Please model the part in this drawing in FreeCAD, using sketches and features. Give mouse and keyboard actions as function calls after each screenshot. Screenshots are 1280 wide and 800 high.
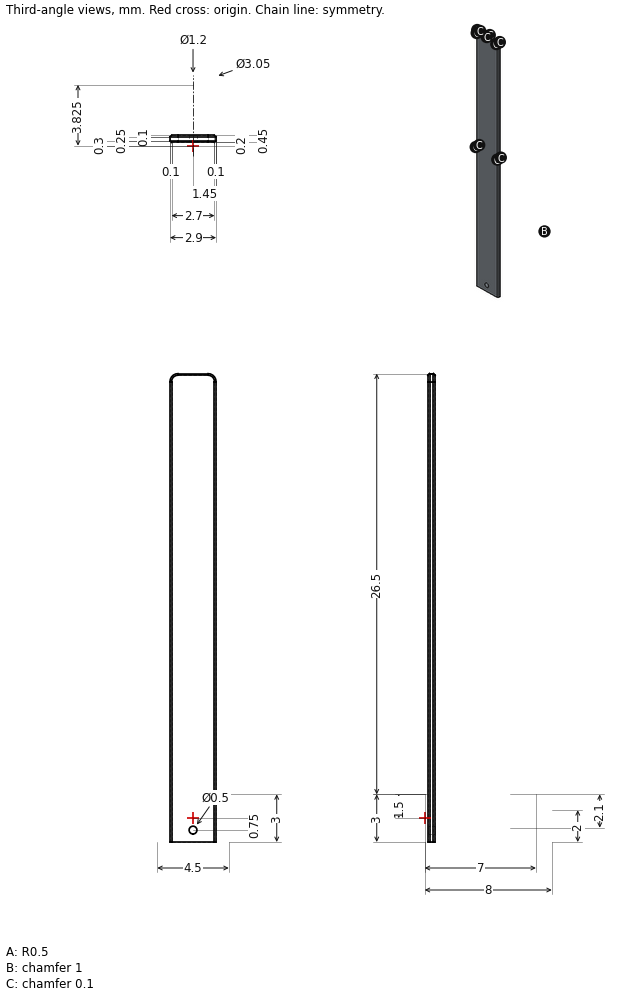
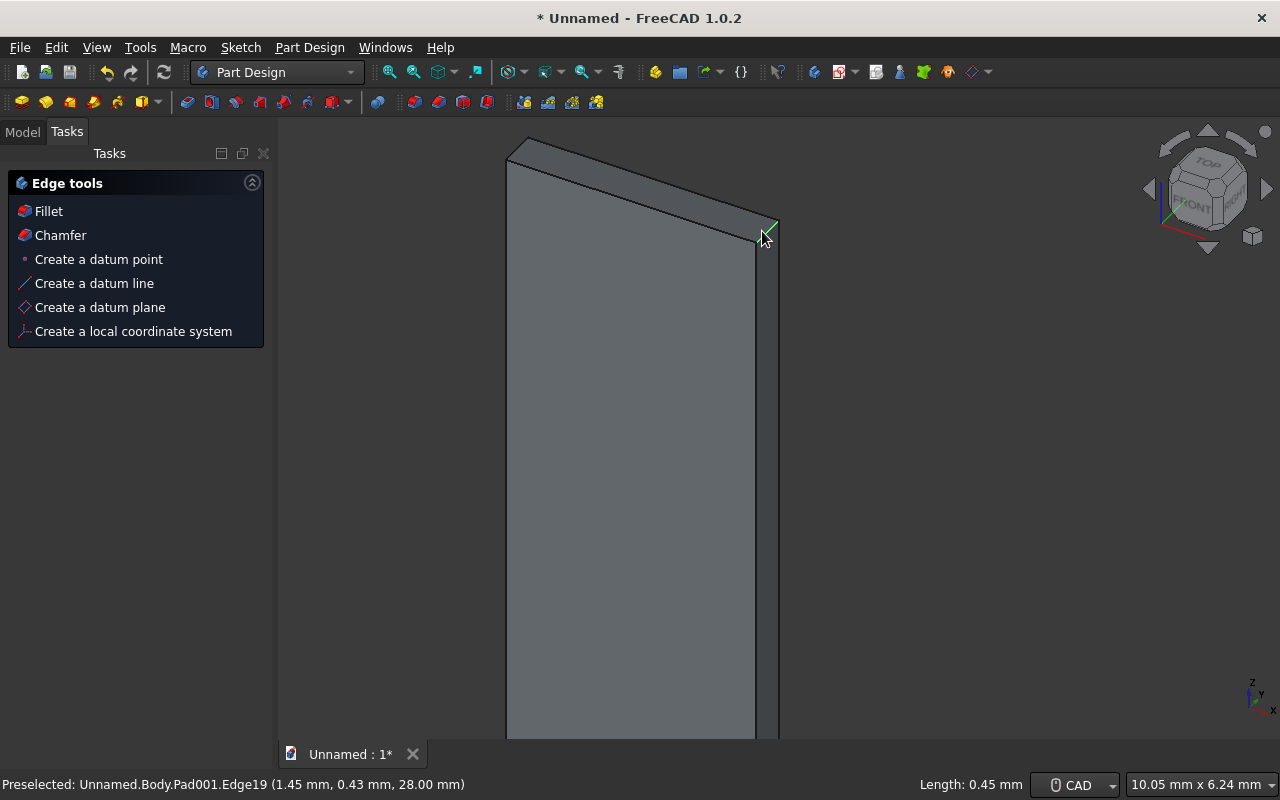
key(v)
key(f)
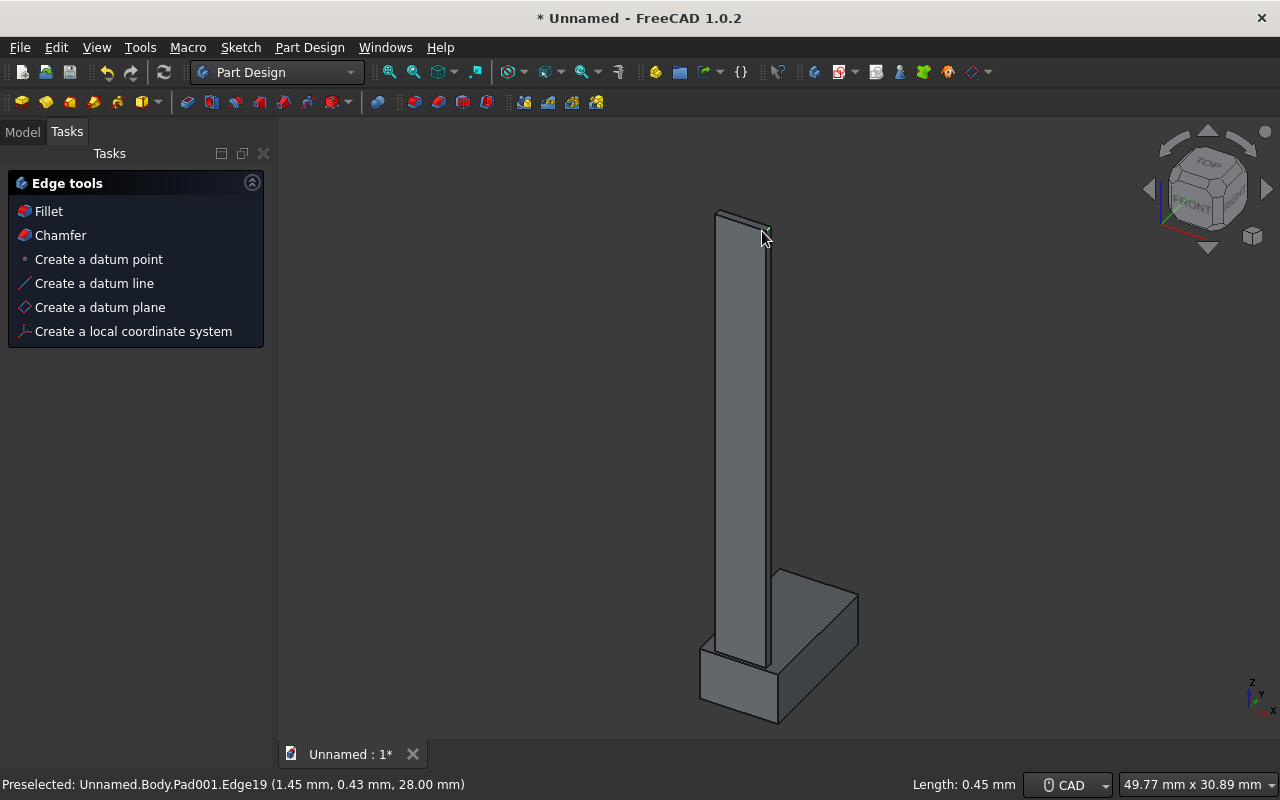
key(0)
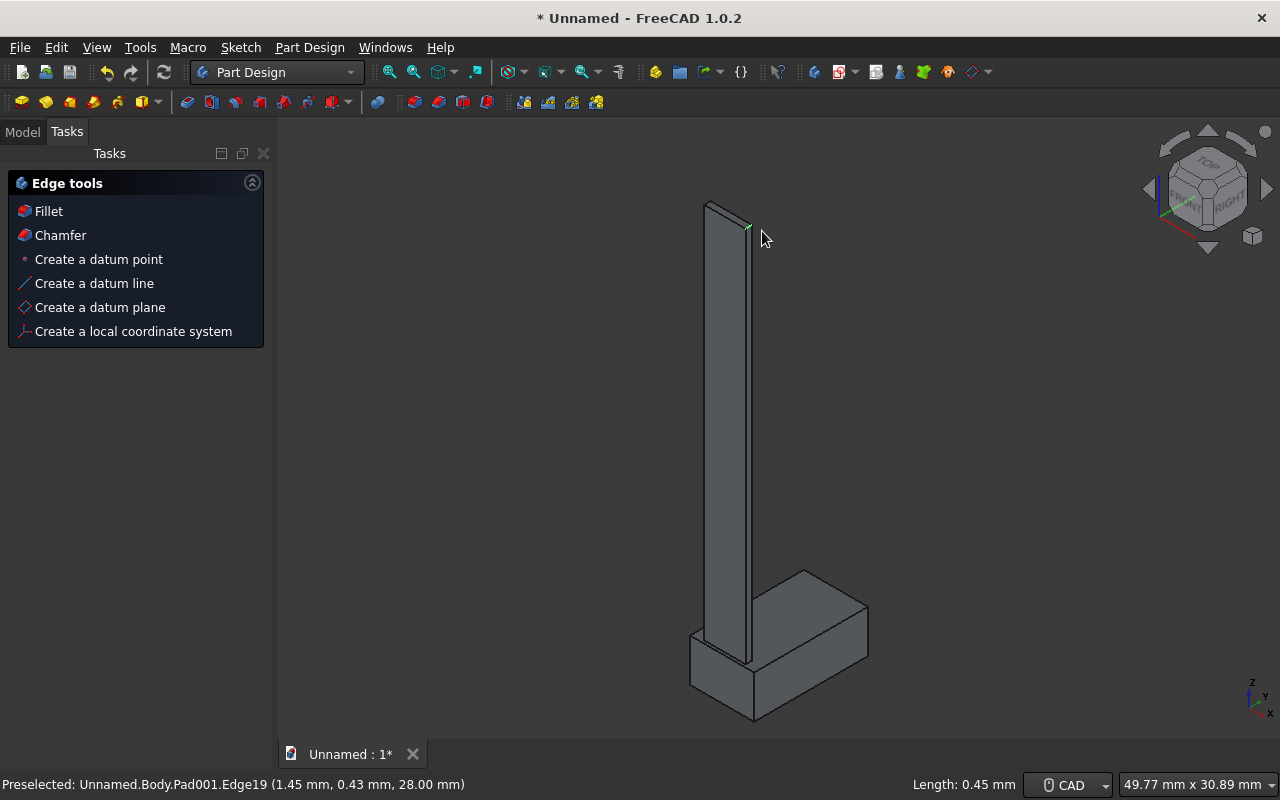
scroll(707, 202, up, 8)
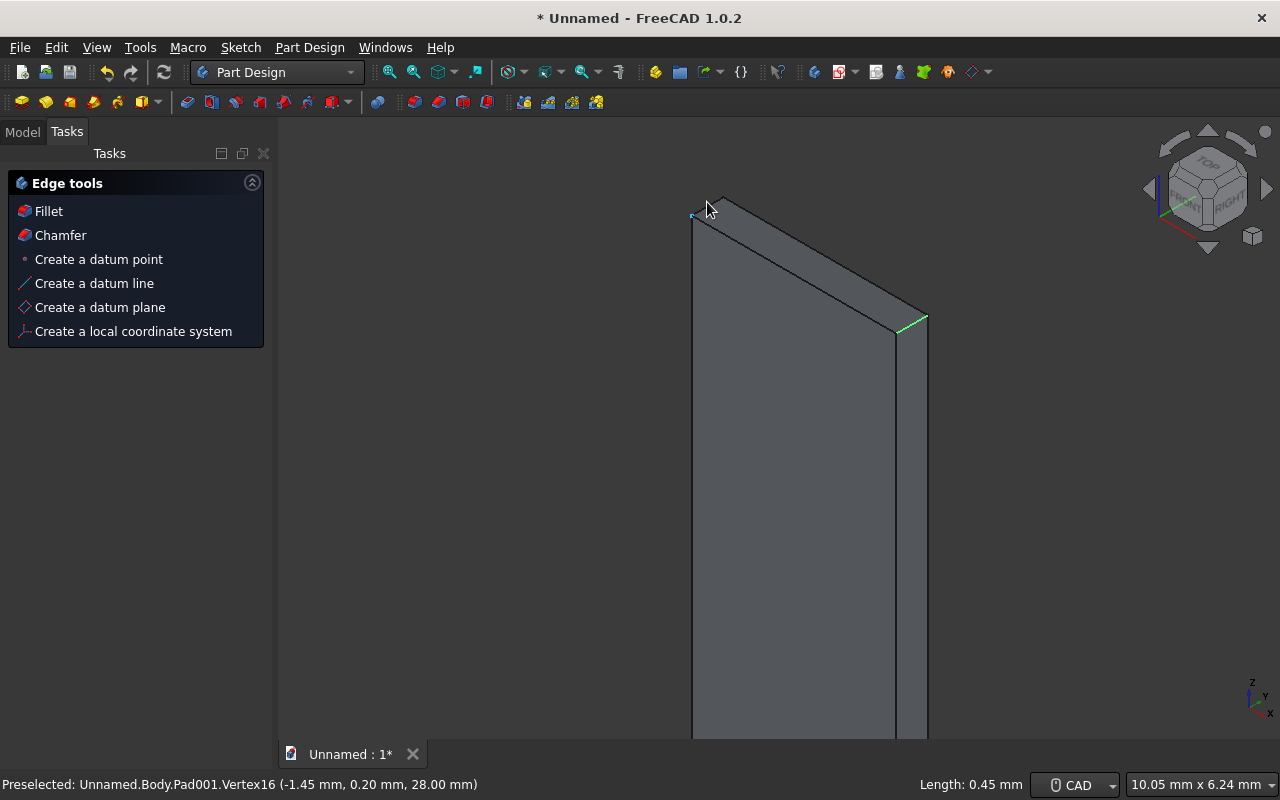
key(v)
key(f)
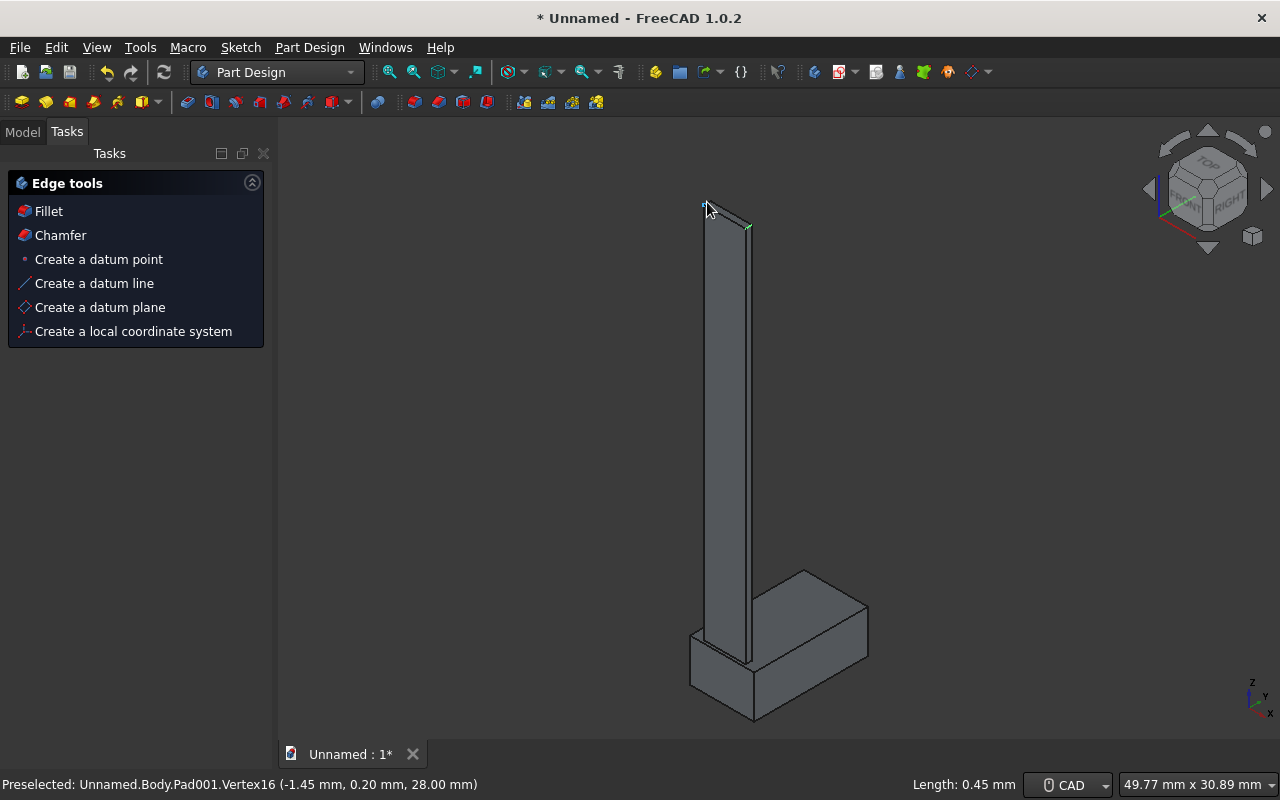
key(2)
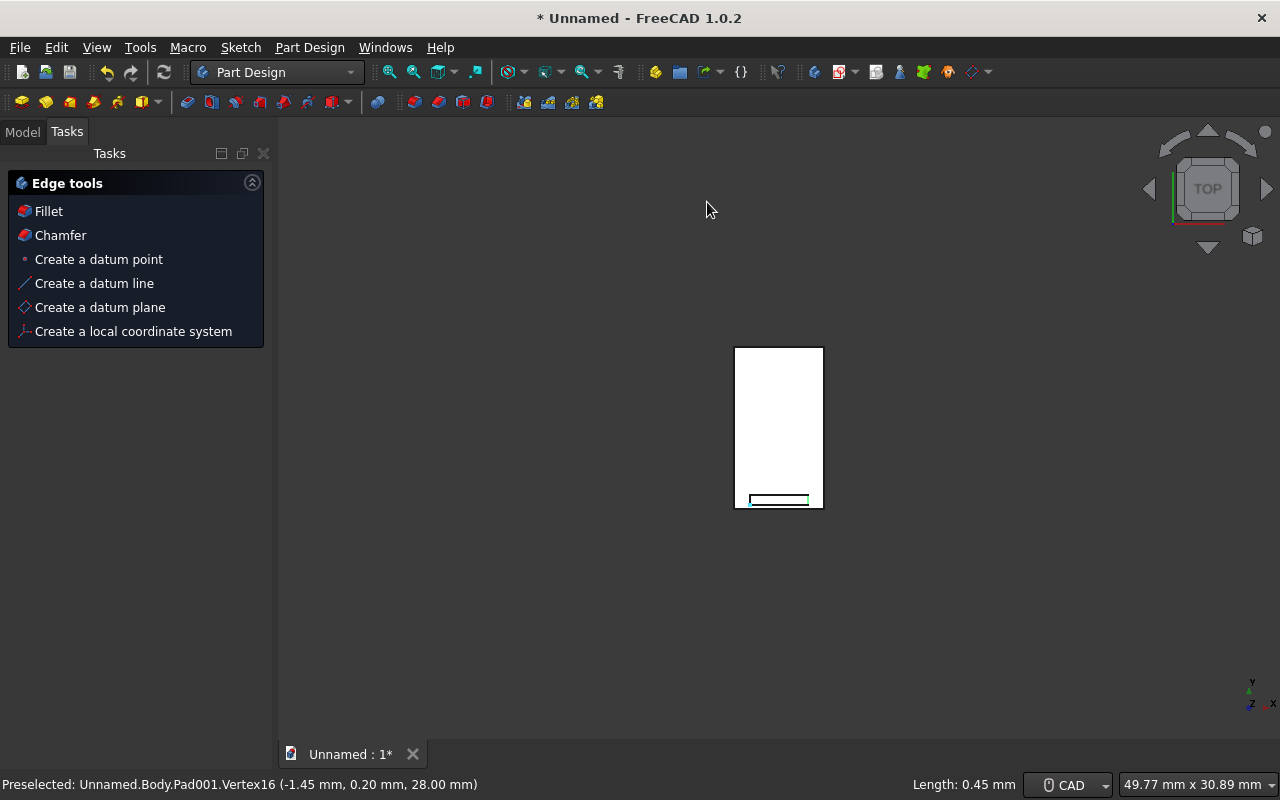
click(390, 72)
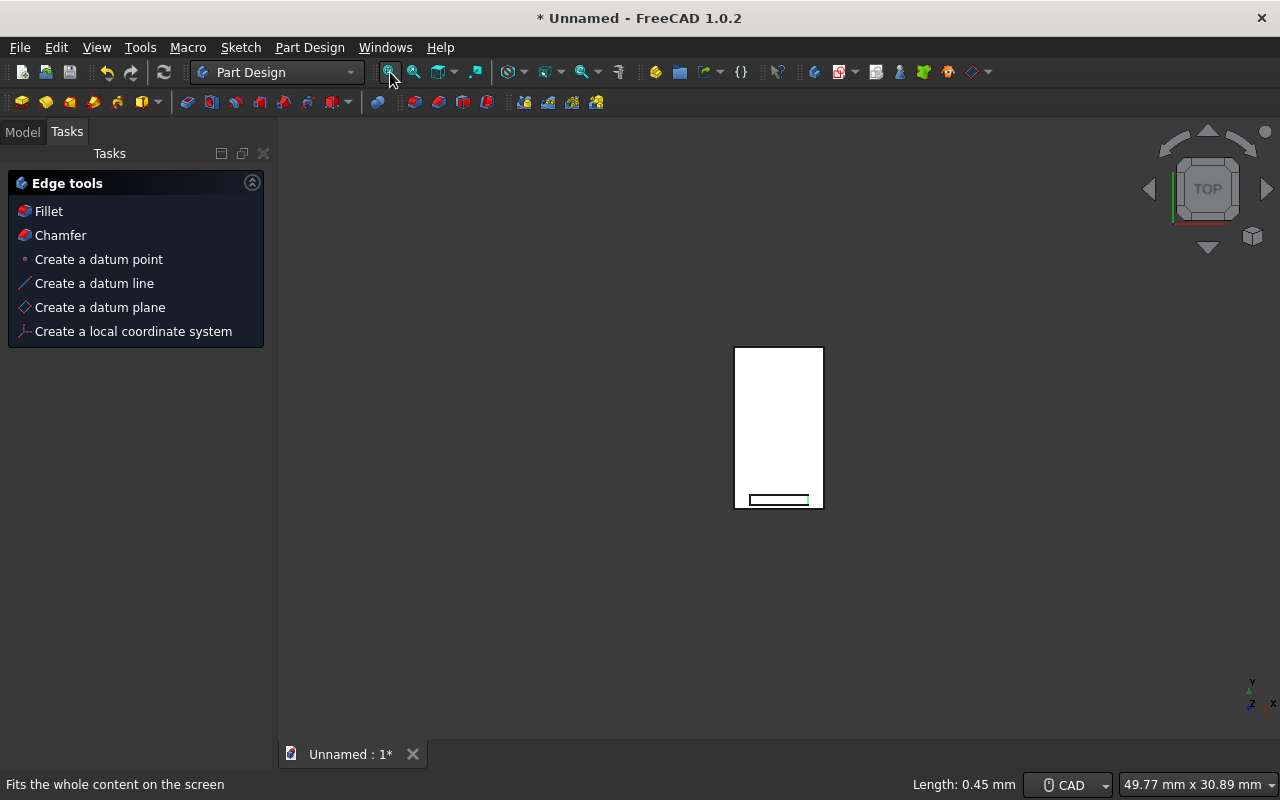
scroll(750, 499, up, 8)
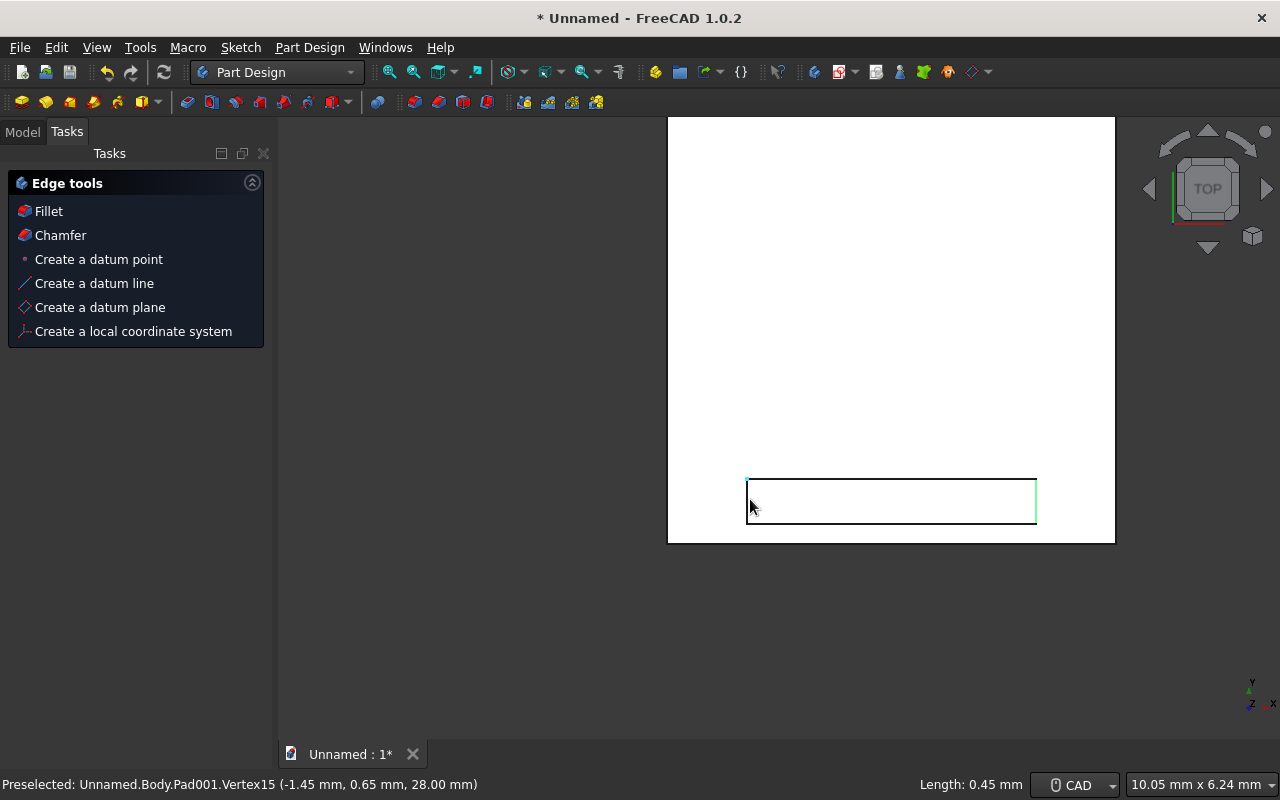
click(747, 500, ctrl)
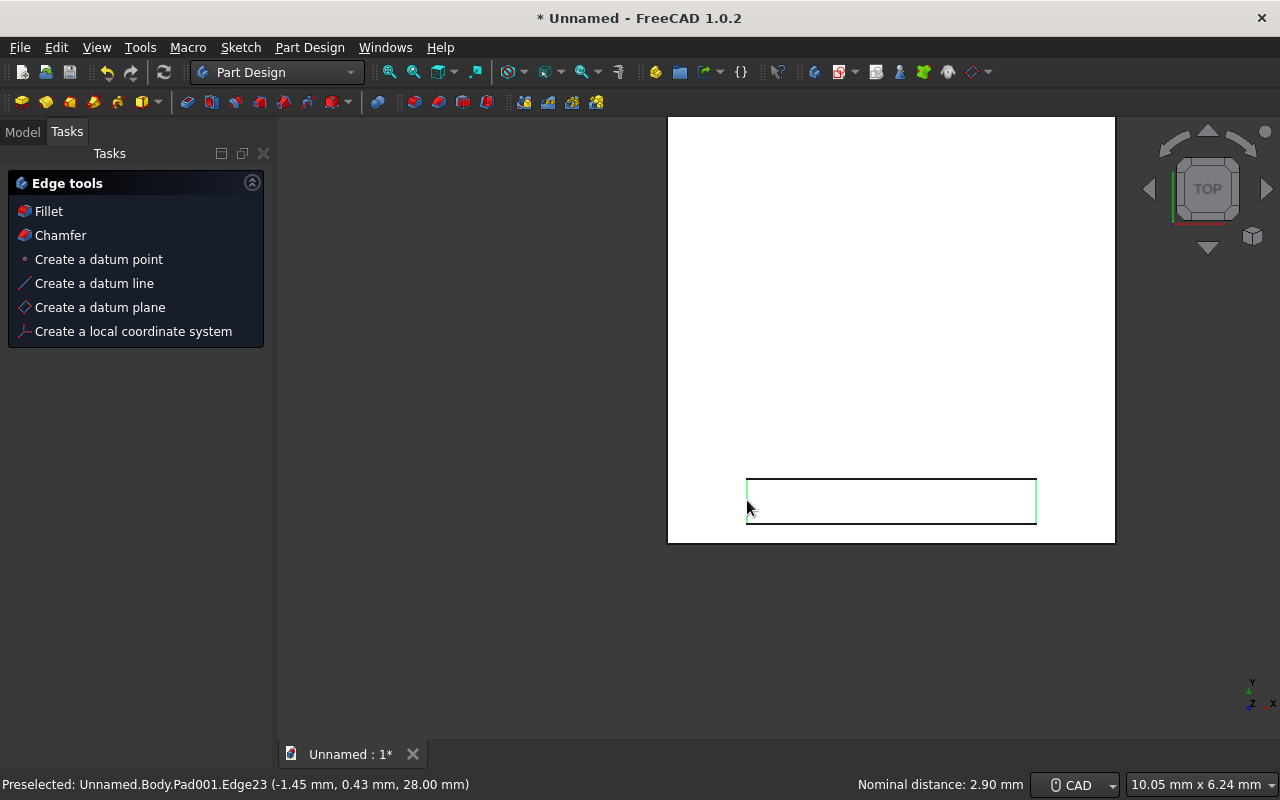
click(416, 102)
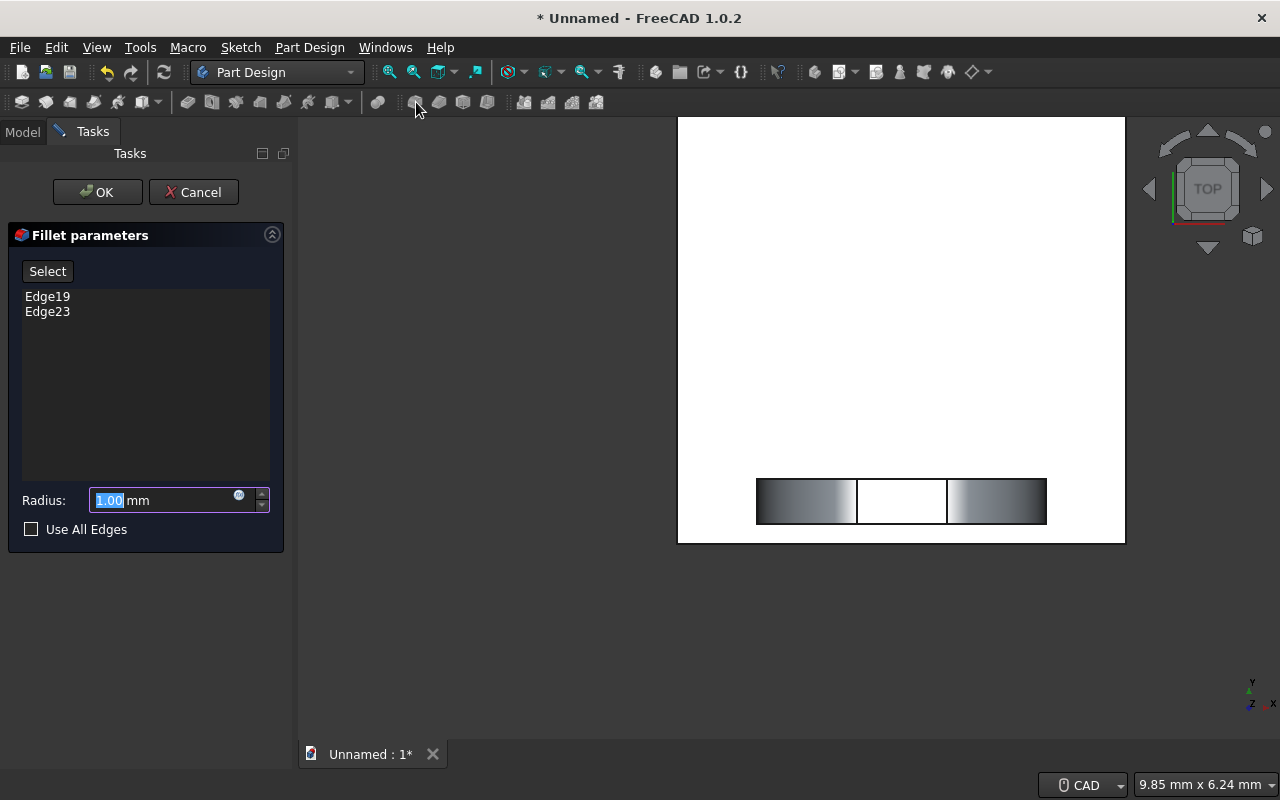
text(0.5)
key(Tab)